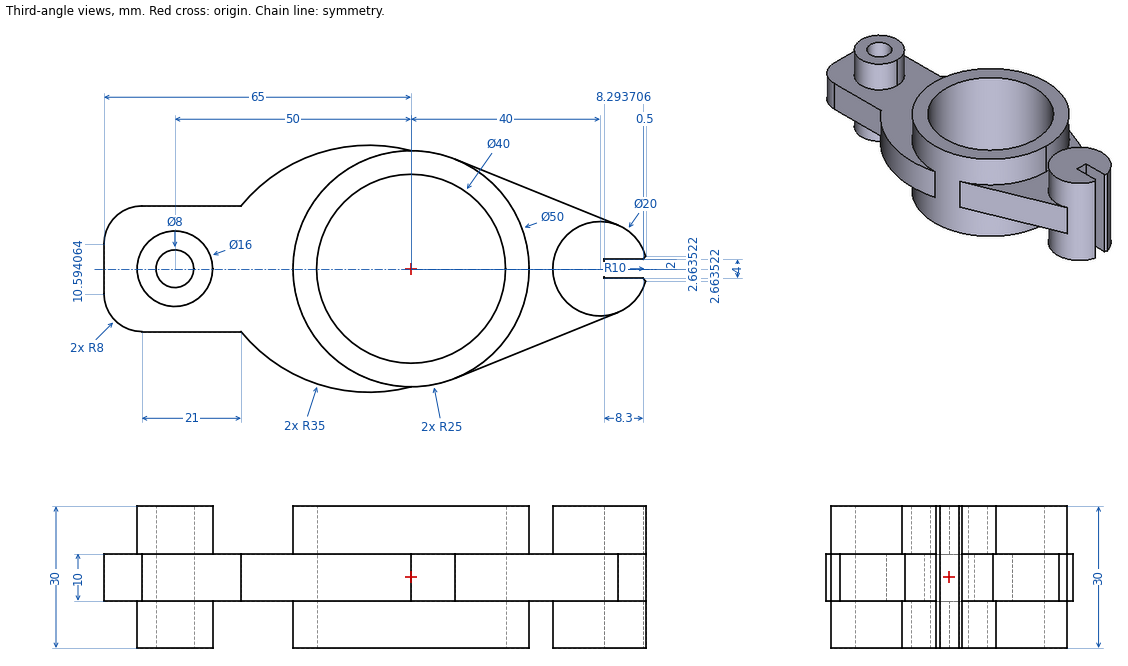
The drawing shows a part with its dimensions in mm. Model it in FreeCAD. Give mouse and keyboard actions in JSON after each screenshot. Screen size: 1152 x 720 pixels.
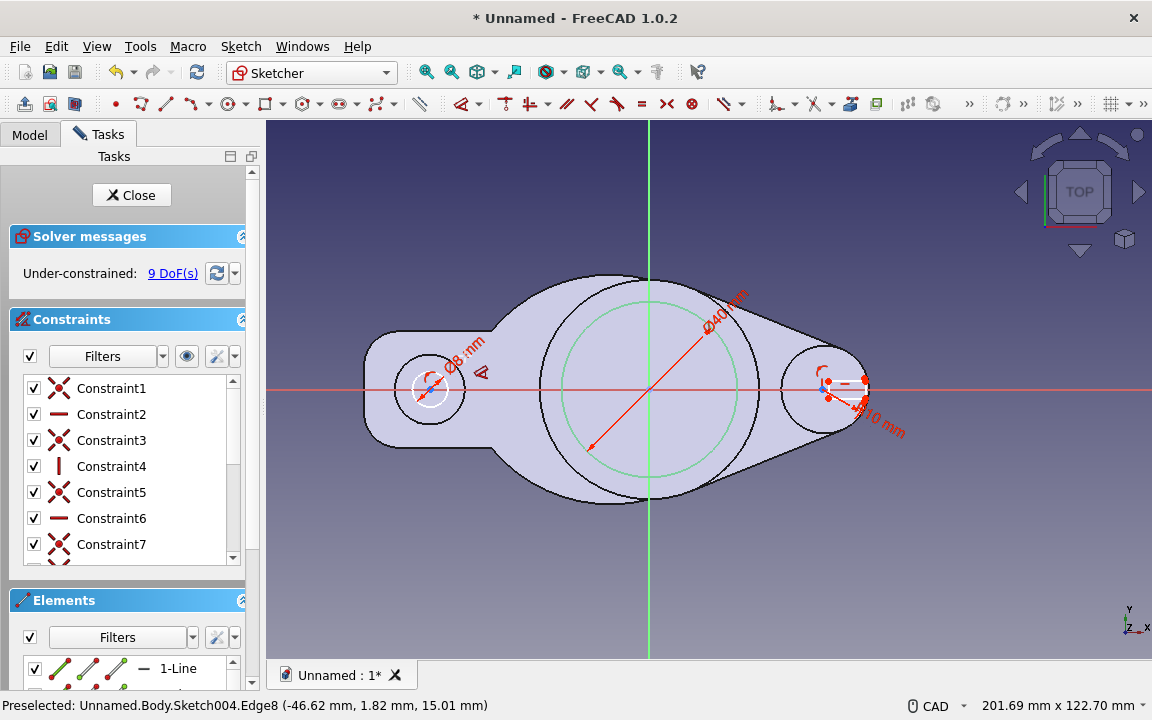
{"action": "scroll", "coordinate": [829, 390], "scroll_direction": "up", "scroll_amount": 5}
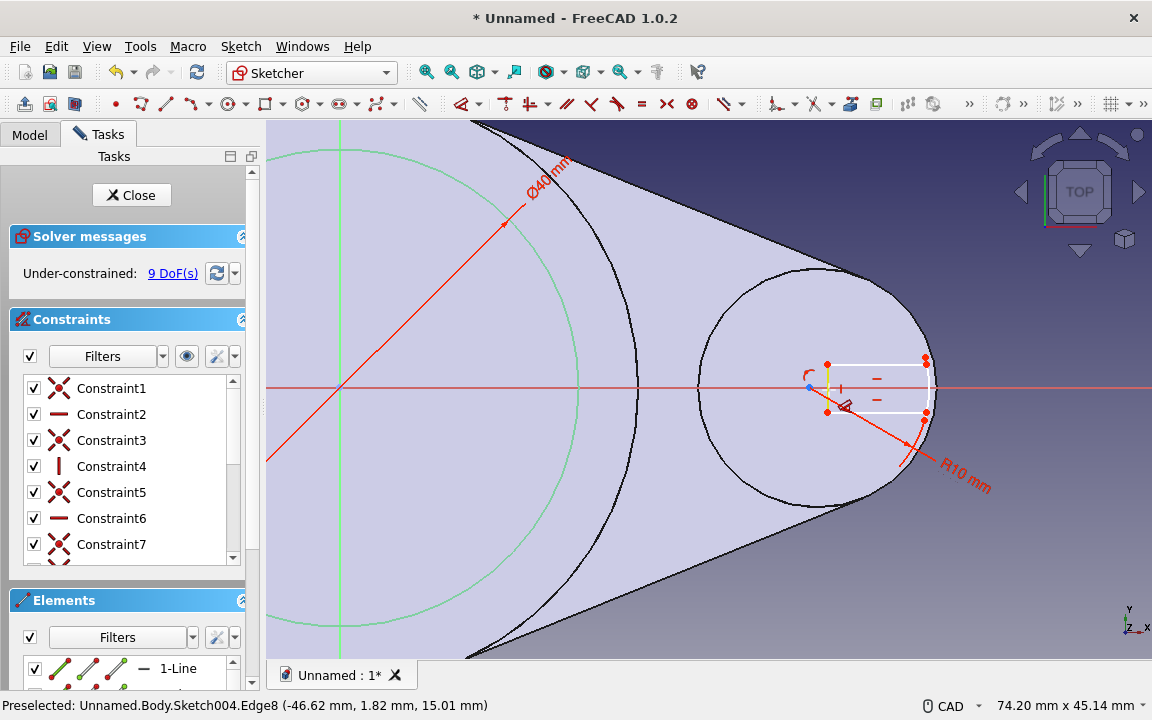
{"action": "left_click", "coordinate": [828, 389]}
{"action": "left_click", "coordinate": [794, 372]}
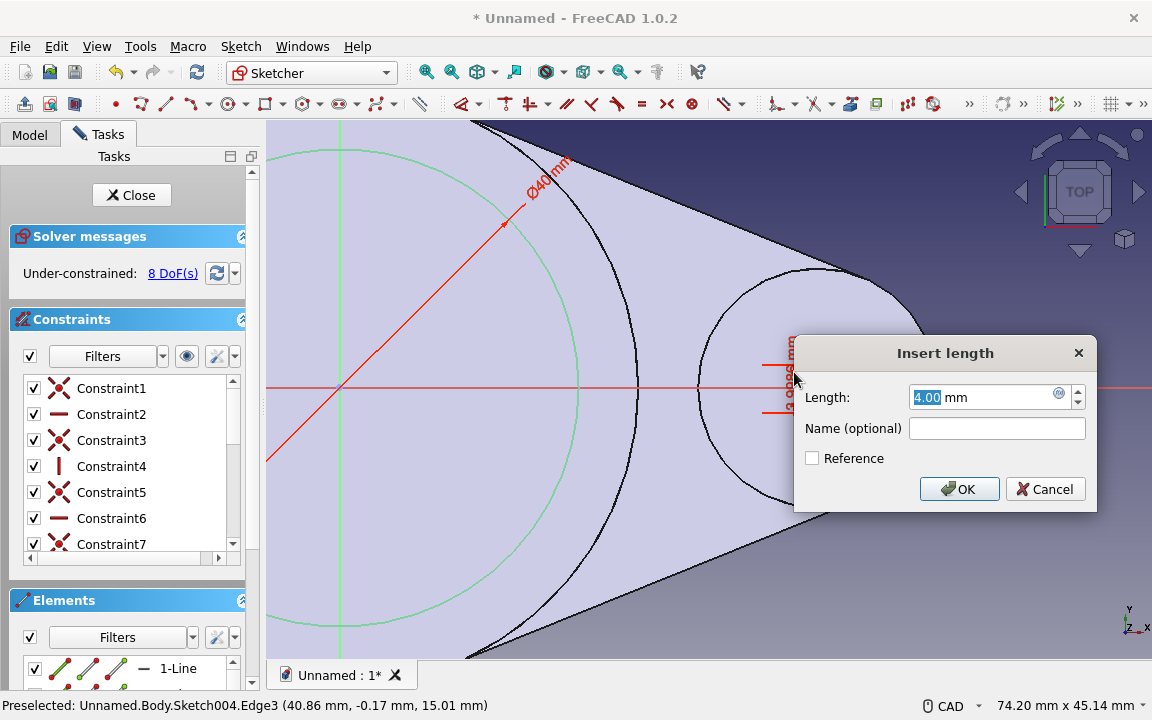
{"action": "type", "text": "4"}
{"action": "key", "text": "Return"}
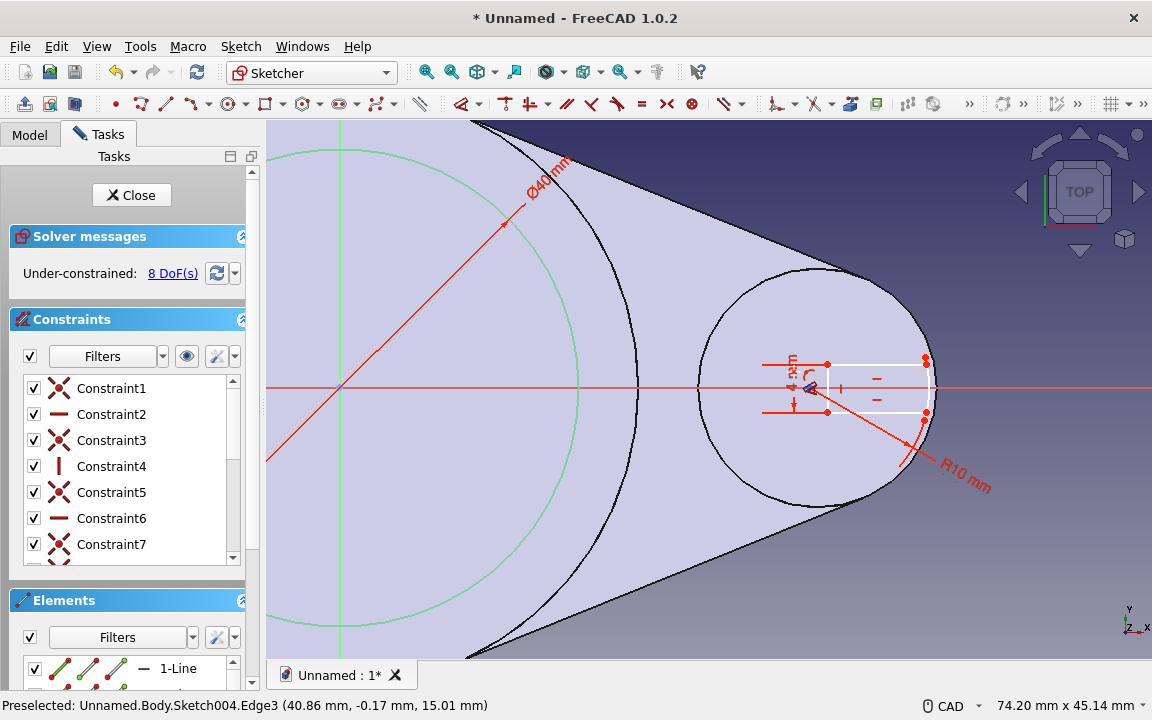
{"action": "scroll", "coordinate": [927, 365], "scroll_direction": "up", "scroll_amount": 3}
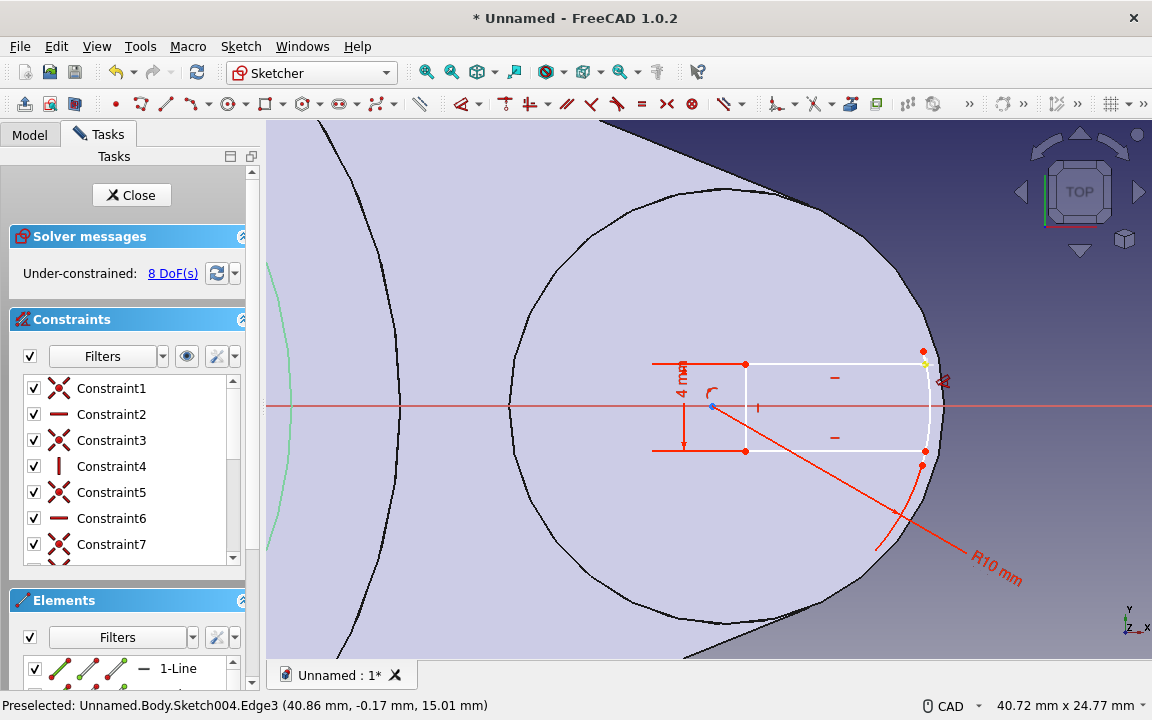
{"action": "left_click", "coordinate": [926, 364]}
{"action": "left_click", "coordinate": [960, 385]}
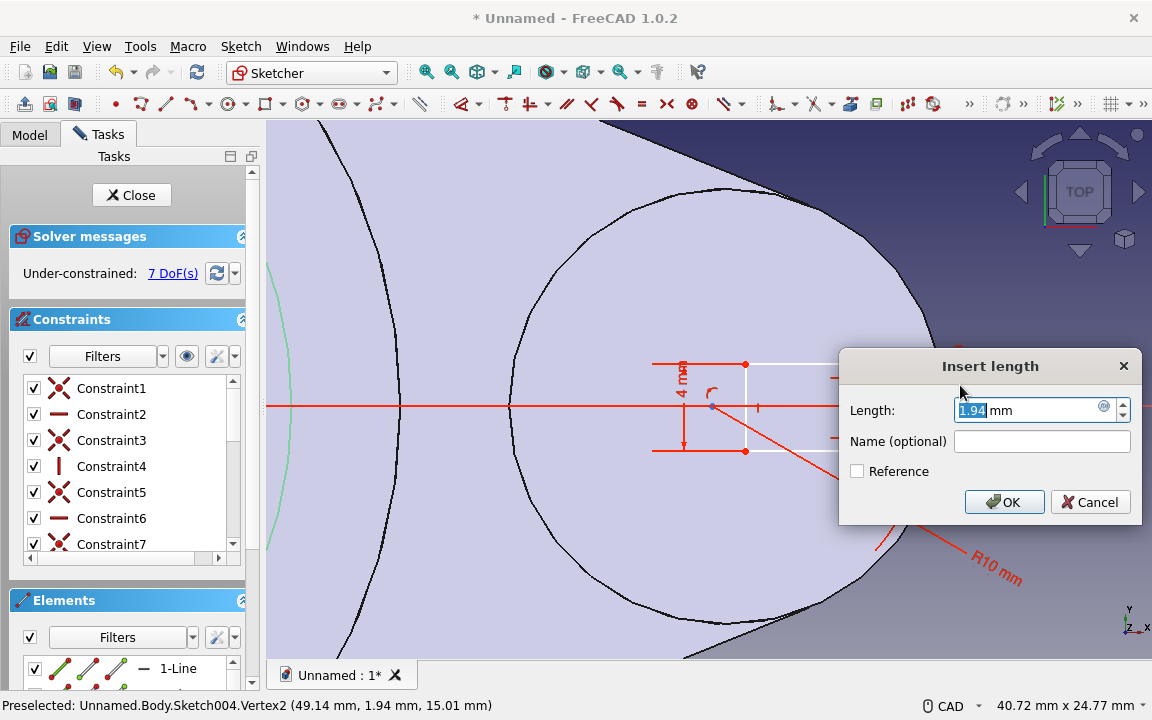
{"action": "type", "text": "2"}
{"action": "key", "text": "Return"}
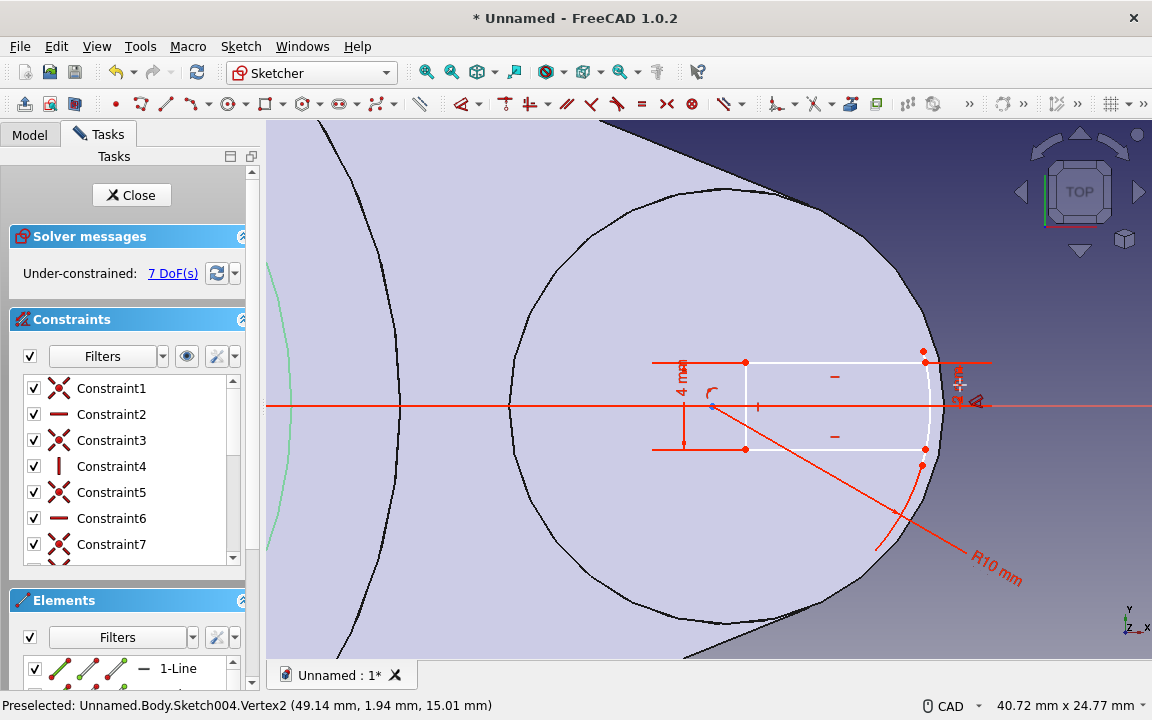
{"action": "scroll", "coordinate": [850, 385], "scroll_direction": "down", "scroll_amount": 8}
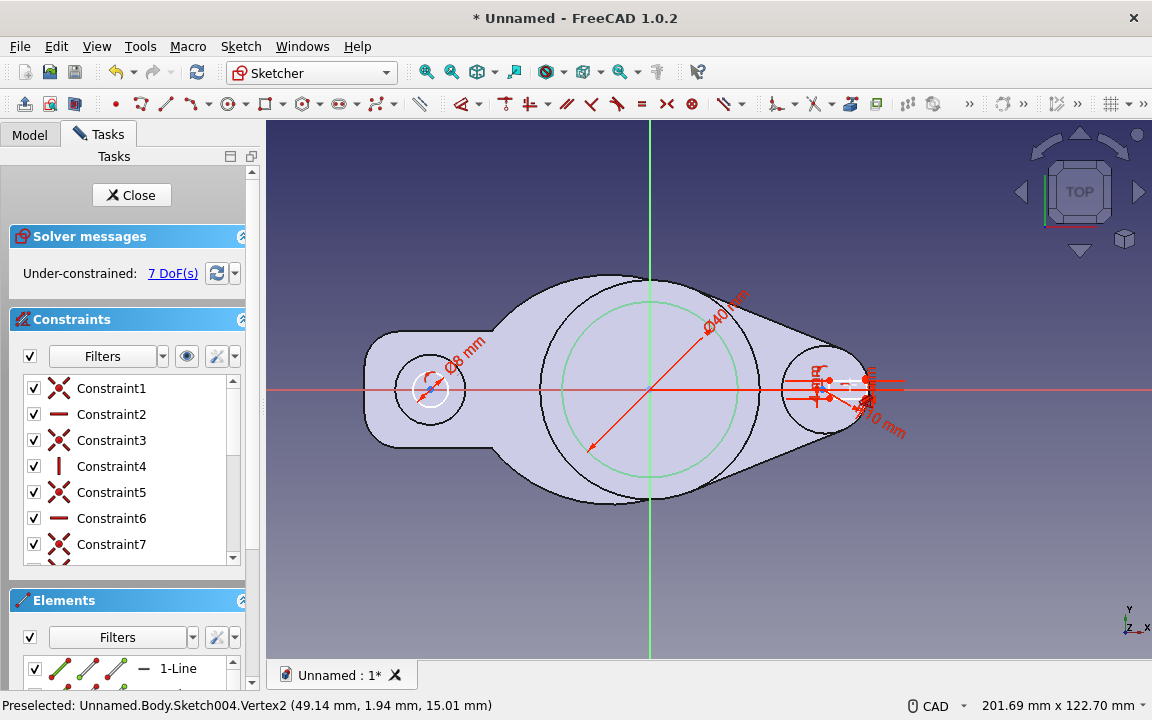
{"action": "left_click", "coordinate": [431, 390]}
{"action": "left_click", "coordinate": [540, 424]}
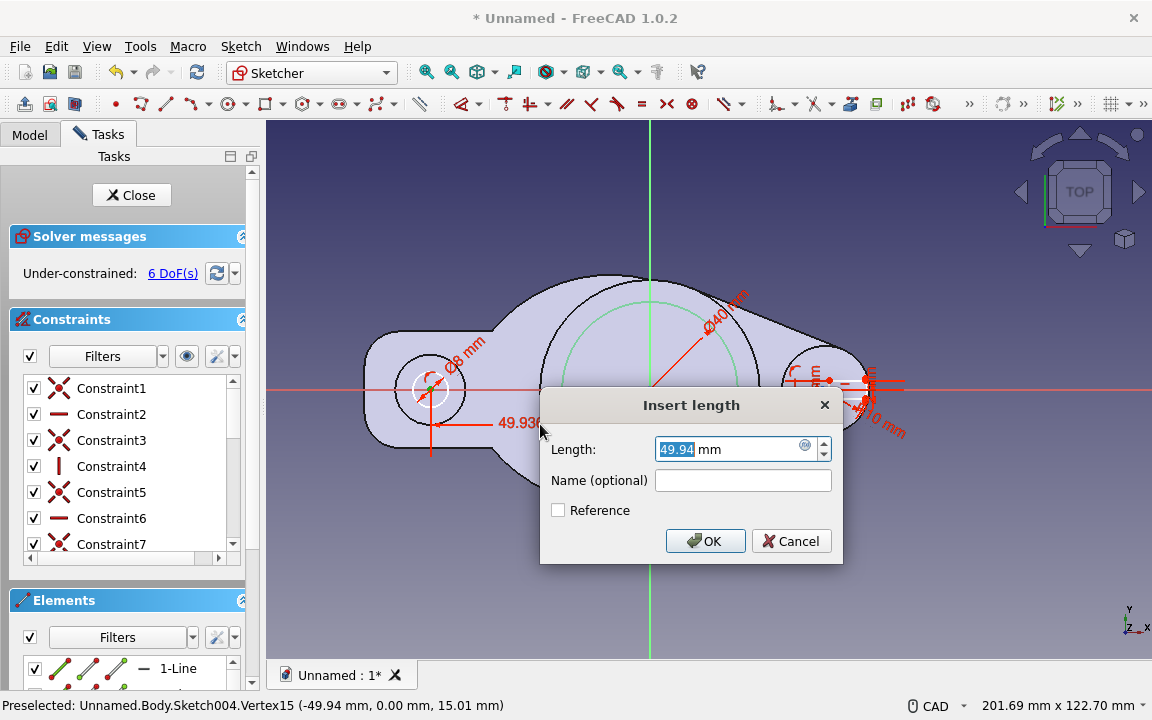
{"action": "type", "text": "50"}
{"action": "key", "text": "Return"}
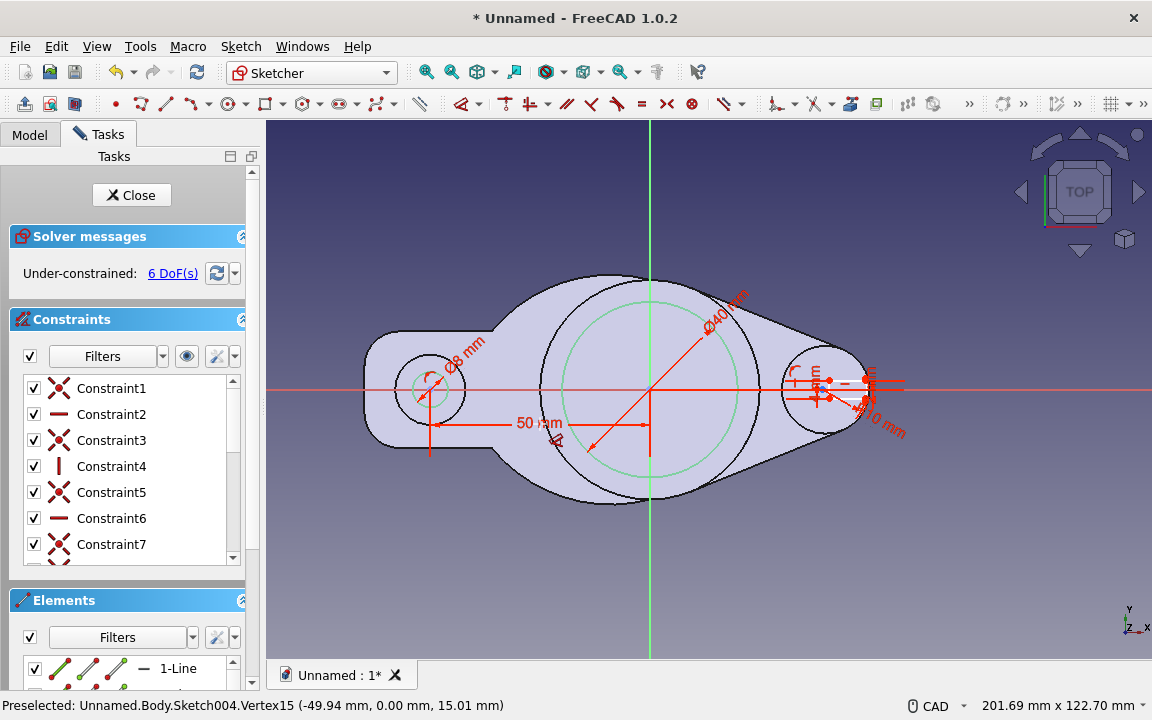
{"action": "scroll", "coordinate": [840, 399], "scroll_direction": "up", "scroll_amount": 3}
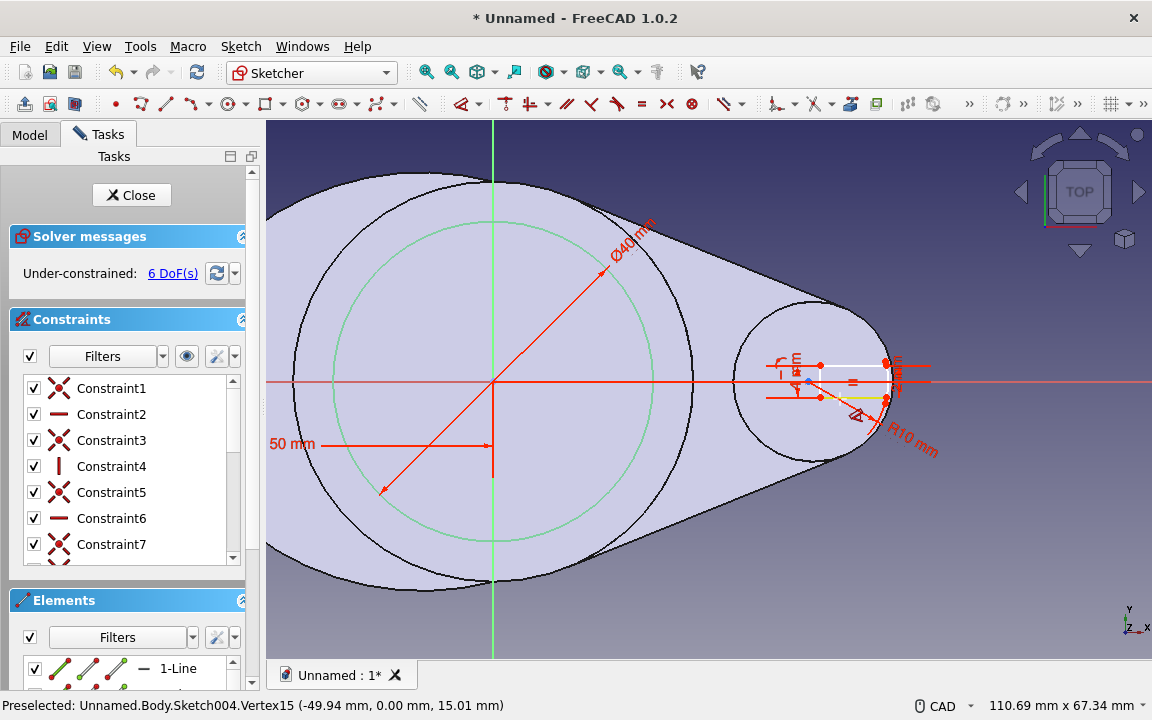
{"action": "left_click", "coordinate": [840, 398]}
{"action": "left_click", "coordinate": [838, 432]}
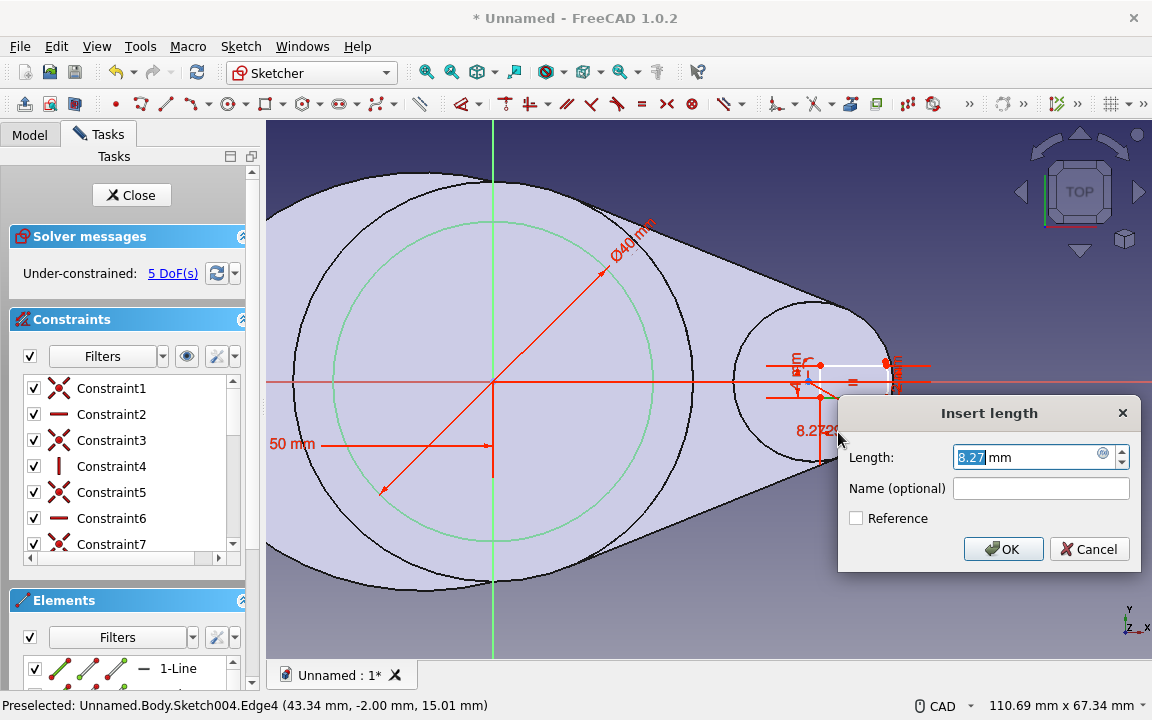
{"action": "type", "text": "8.3"}
{"action": "key", "text": "Return"}